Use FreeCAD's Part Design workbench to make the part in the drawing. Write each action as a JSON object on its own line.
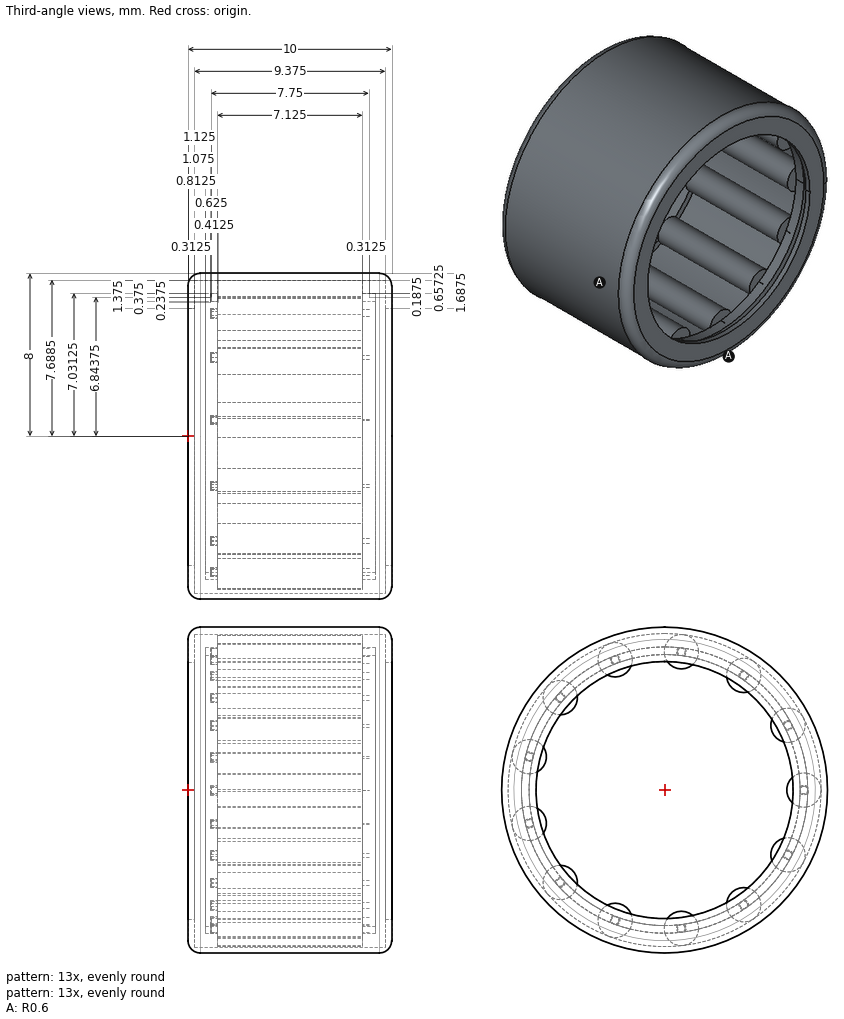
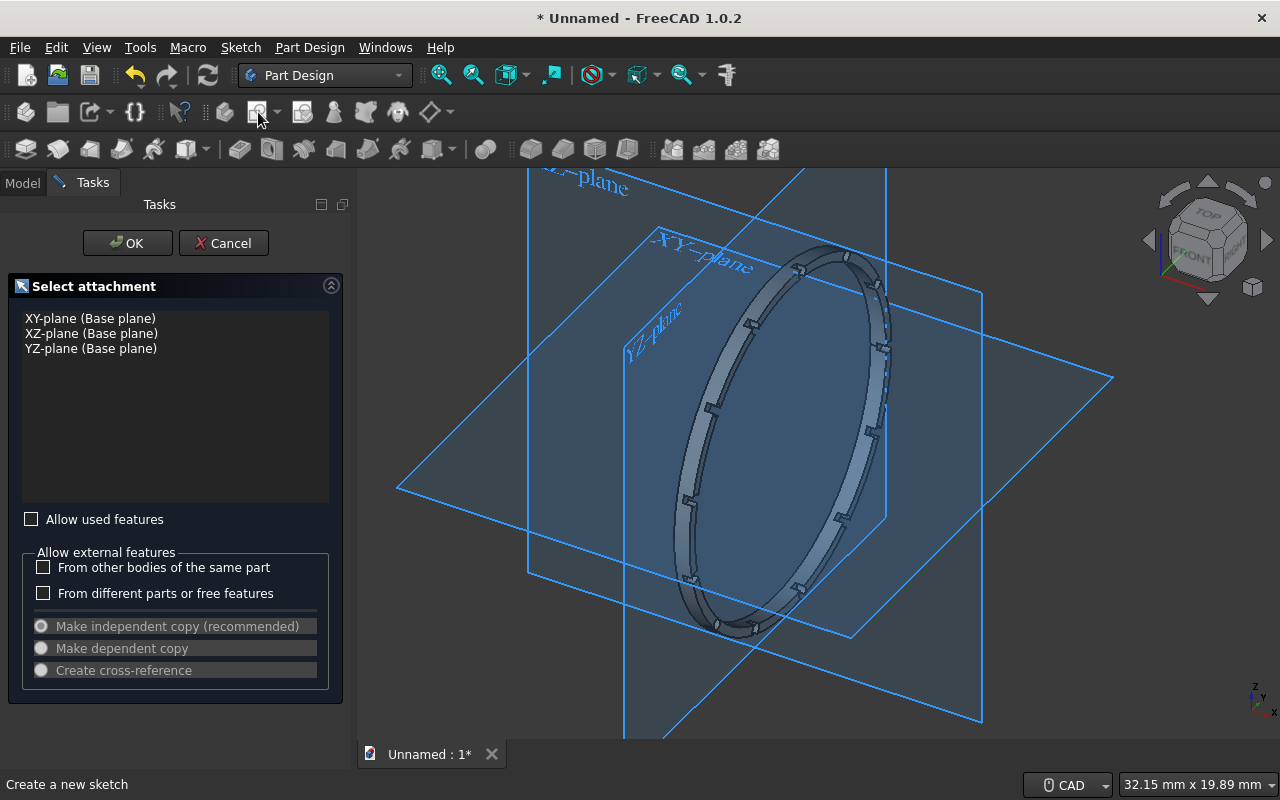
{"action": "left_click", "coordinate": [82, 318]}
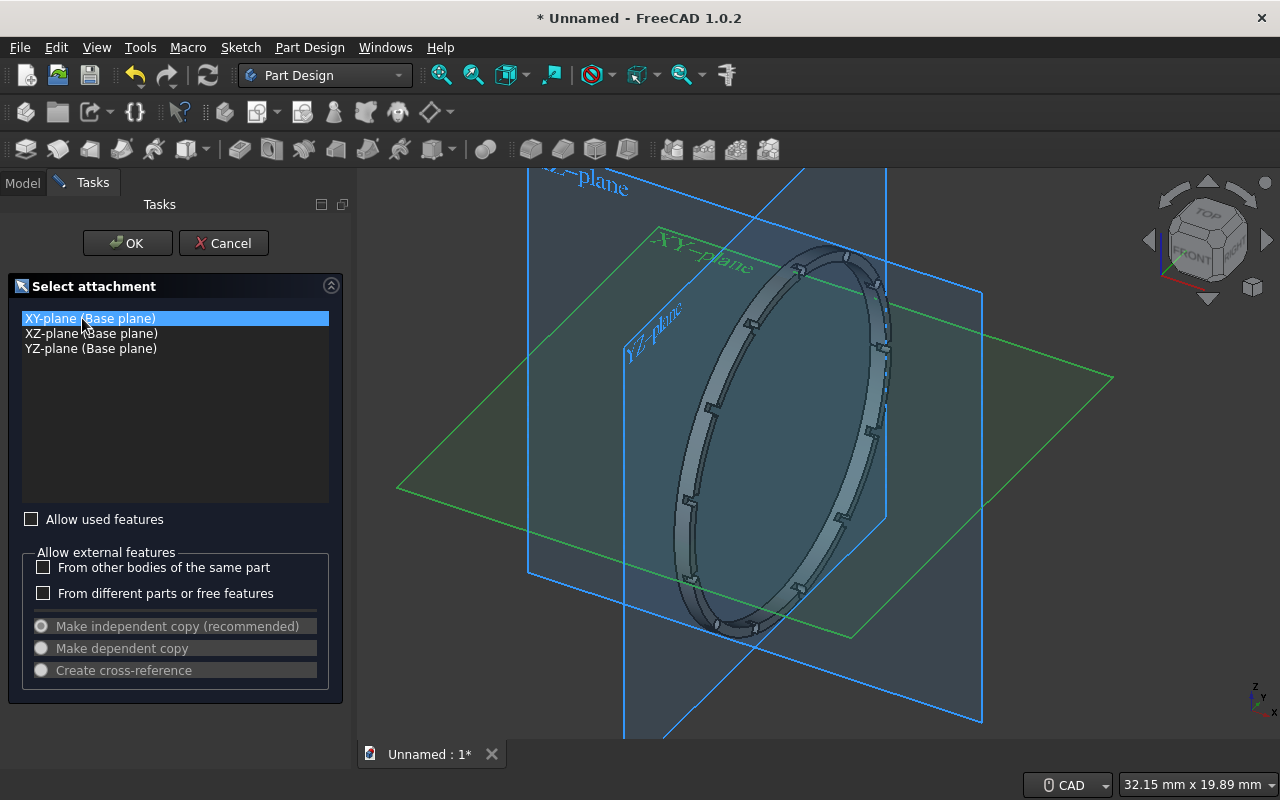
{"action": "left_click", "coordinate": [128, 243]}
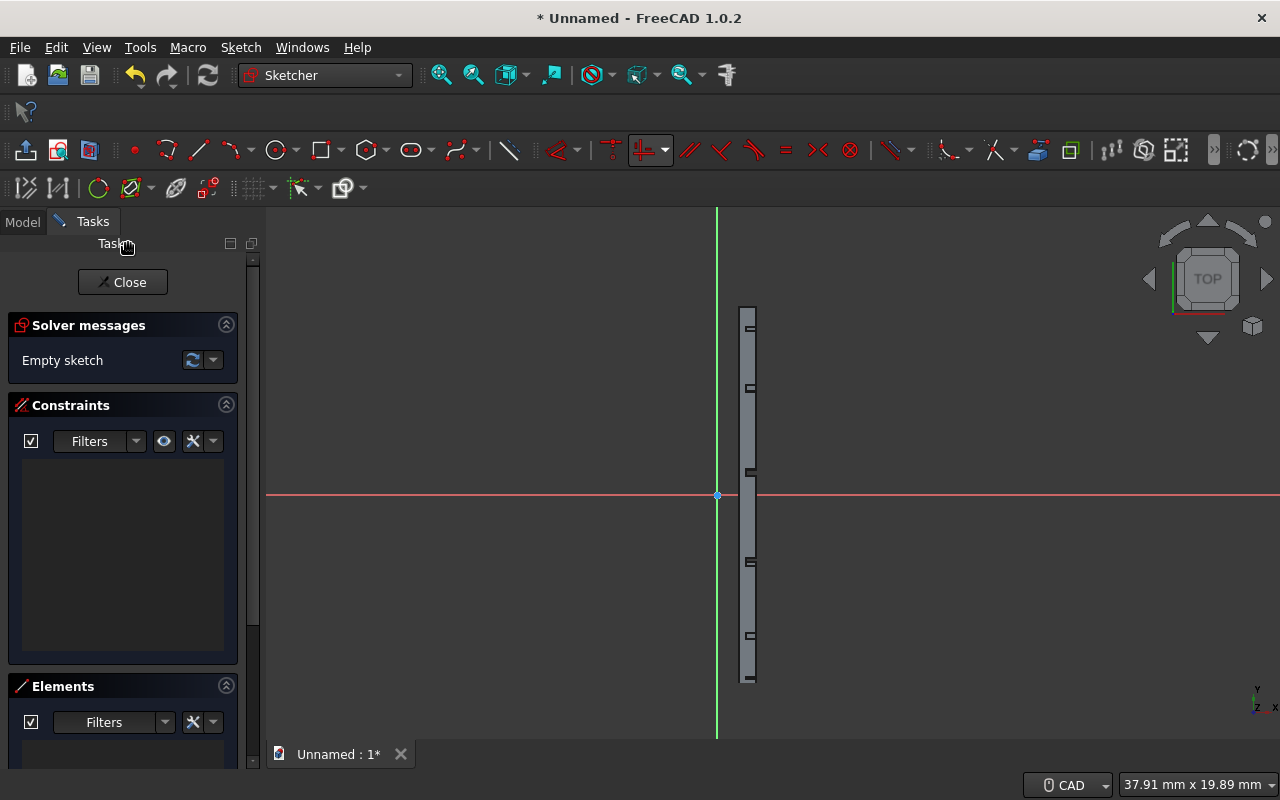
{"action": "left_click", "coordinate": [90, 150]}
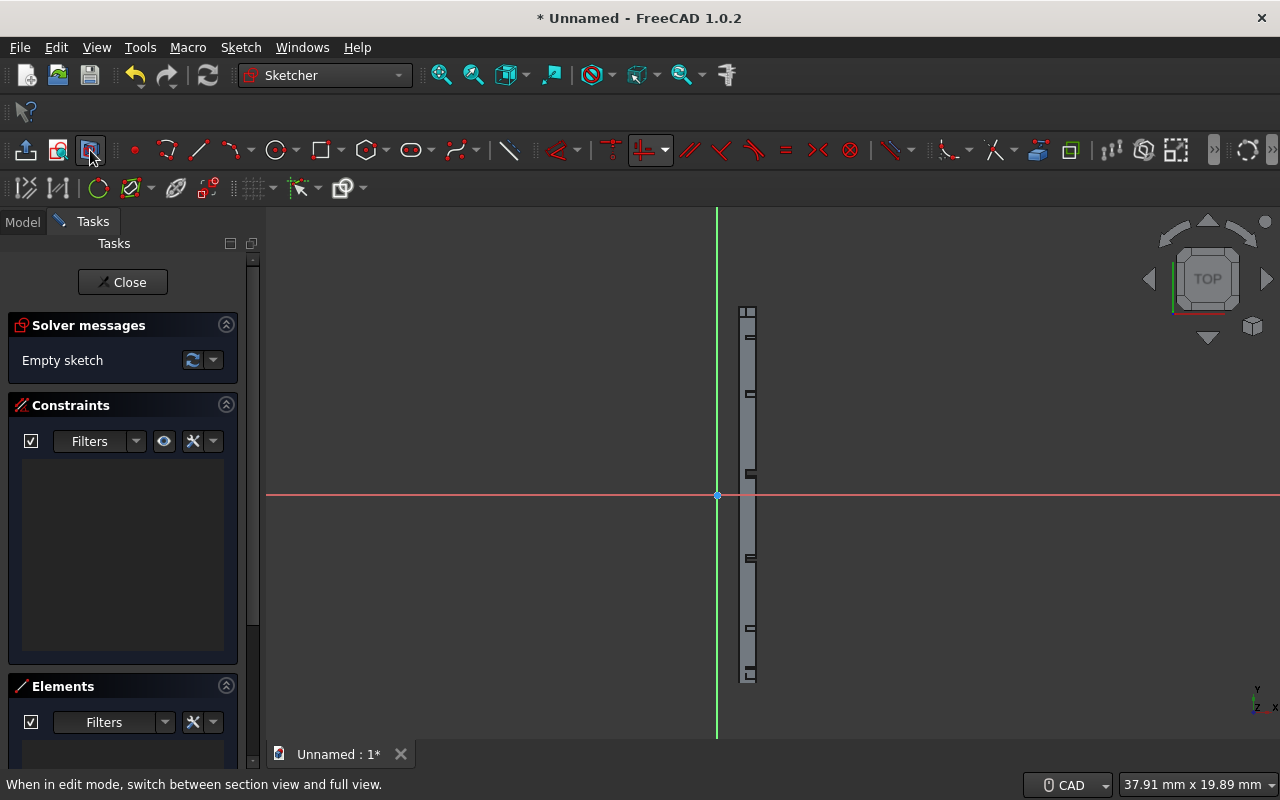
{"action": "scroll", "coordinate": [1115, 235], "scroll_direction": "up", "scroll_amount": 2}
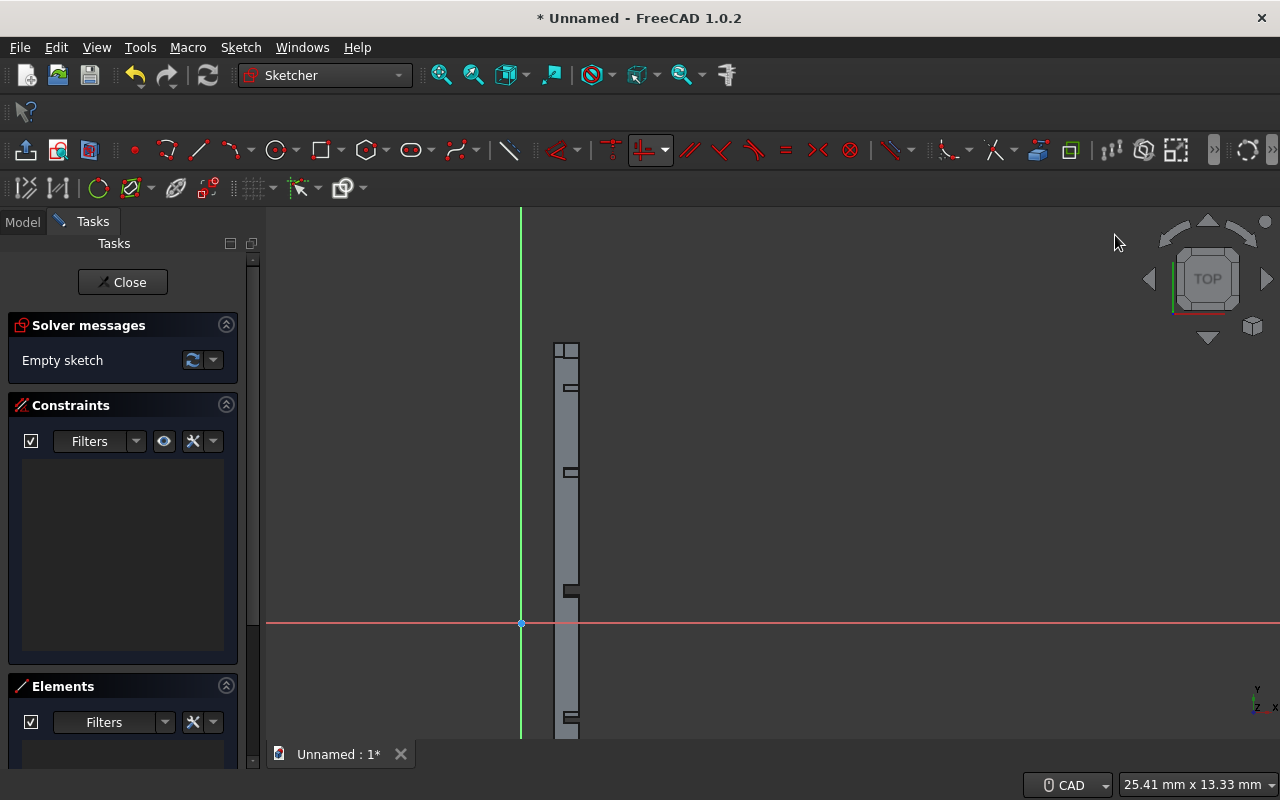
{"action": "left_click", "coordinate": [168, 150]}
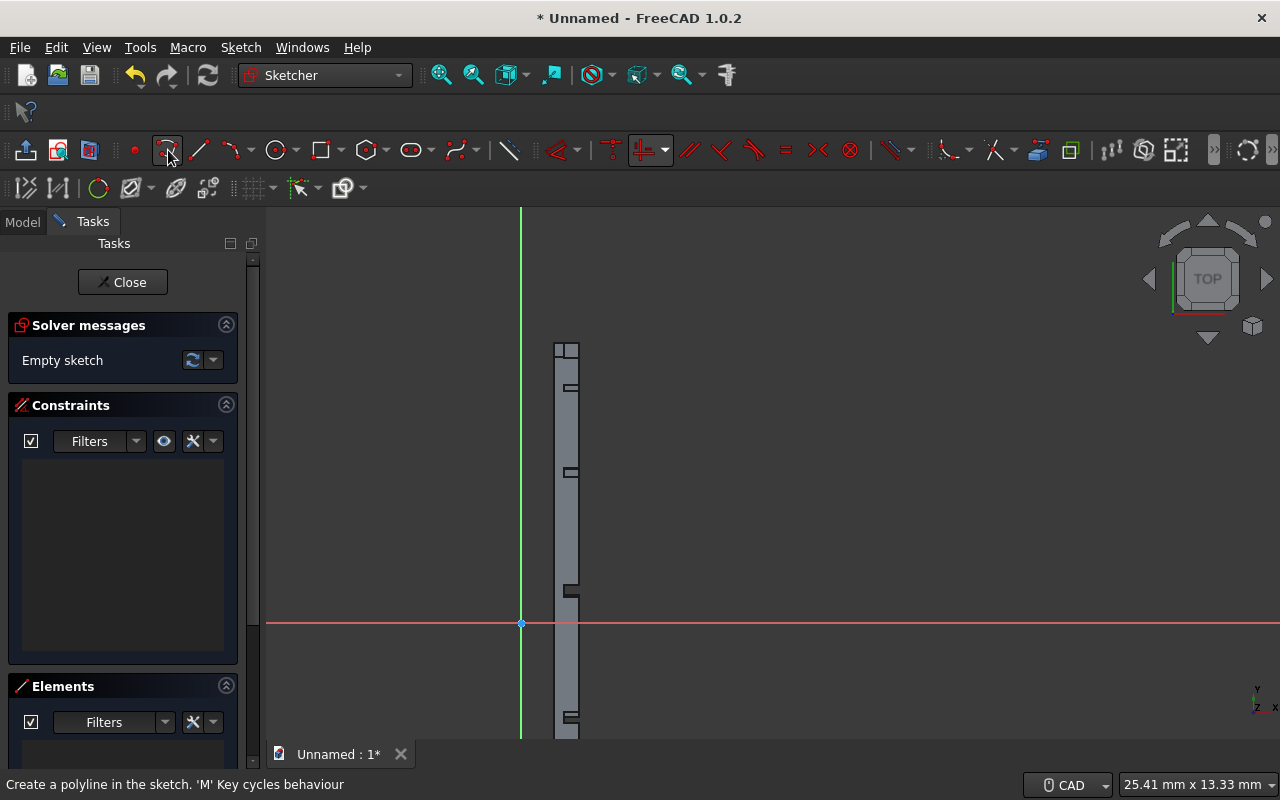
{"action": "left_click", "coordinate": [566, 350]}
{"action": "left_click", "coordinate": [875, 350]}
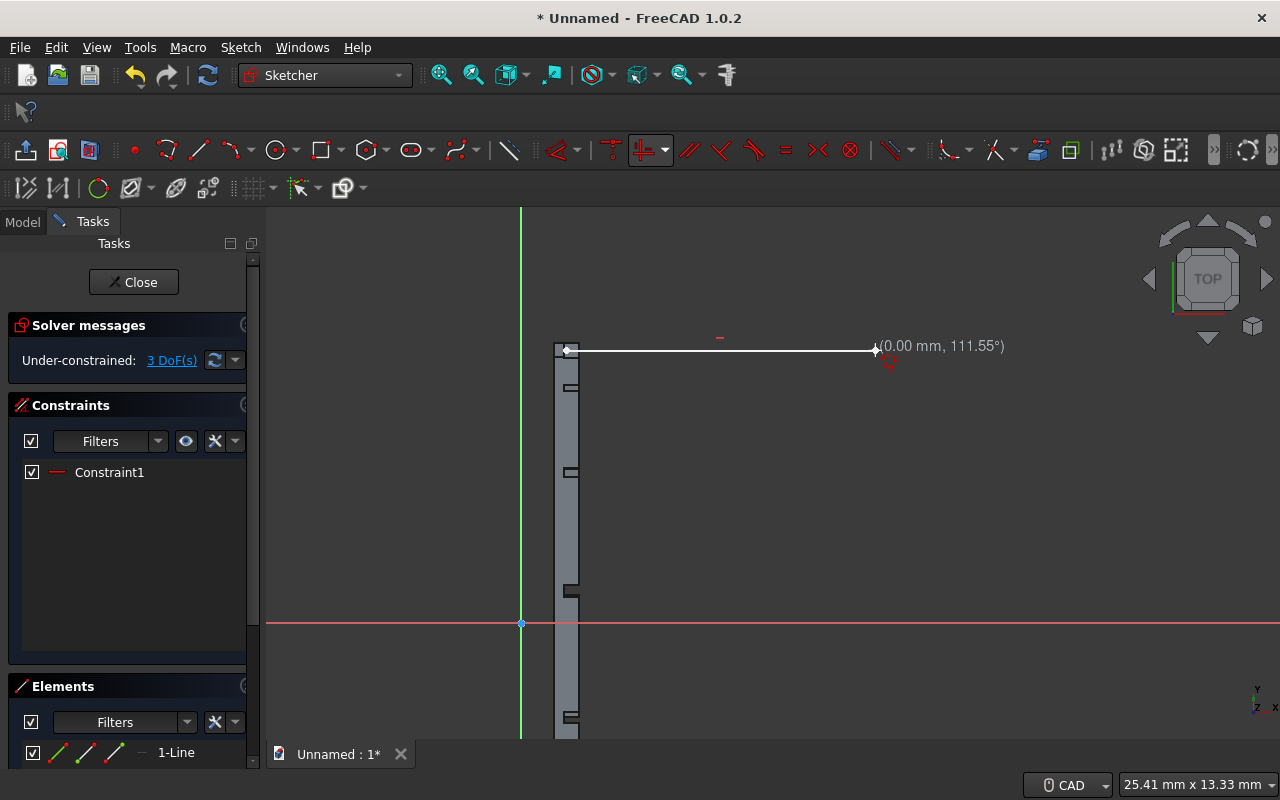
{"action": "scroll", "coordinate": [875, 343], "scroll_direction": "up", "scroll_amount": 4}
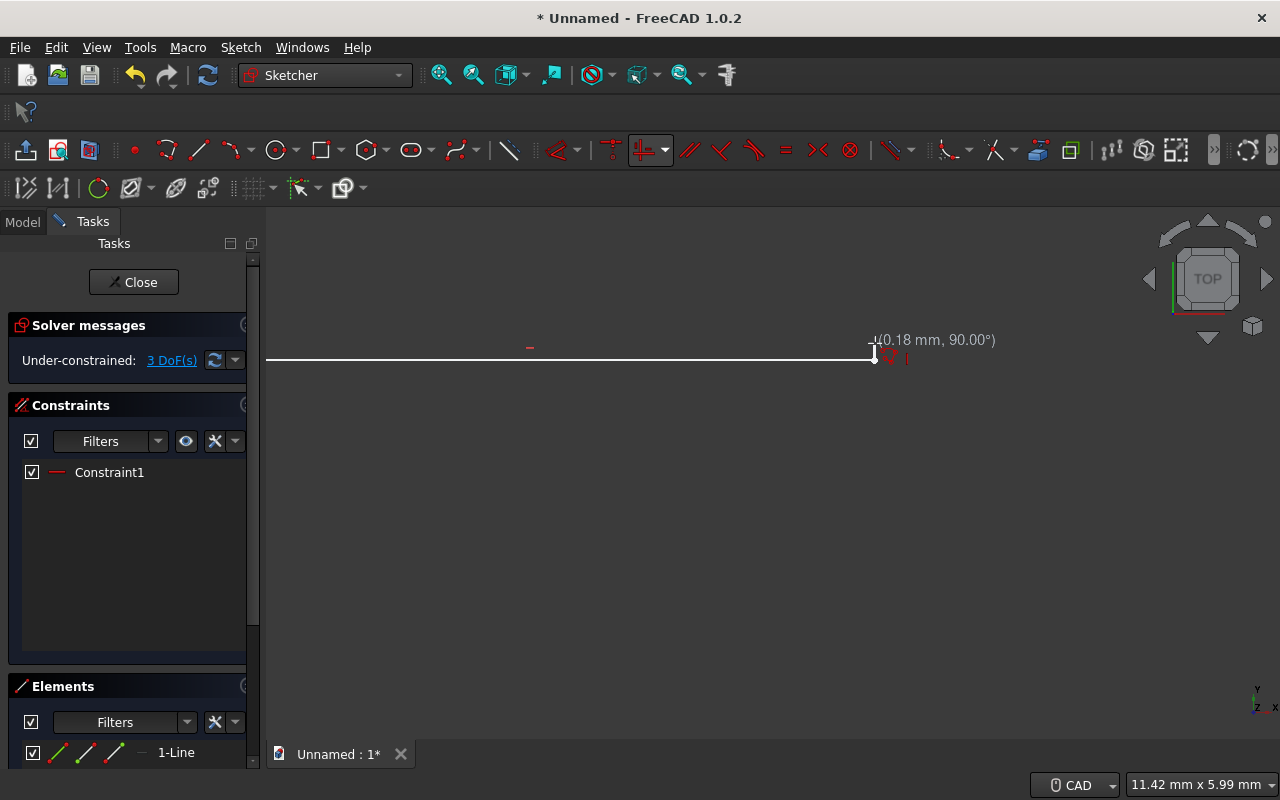
{"action": "left_click", "coordinate": [874, 342]}
{"action": "left_click", "coordinate": [847, 342]}
{"action": "left_click", "coordinate": [847, 283]}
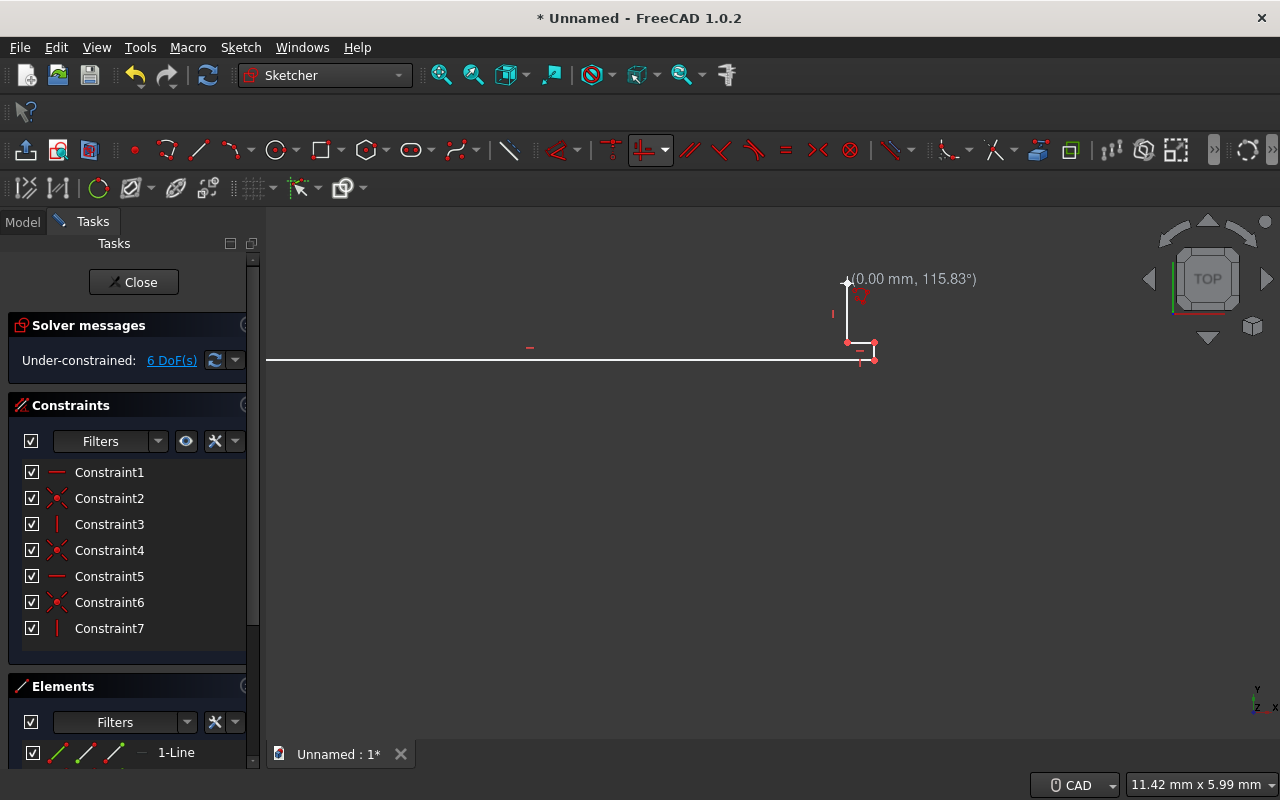
{"action": "scroll", "coordinate": [774, 349], "scroll_direction": "down", "scroll_amount": 4}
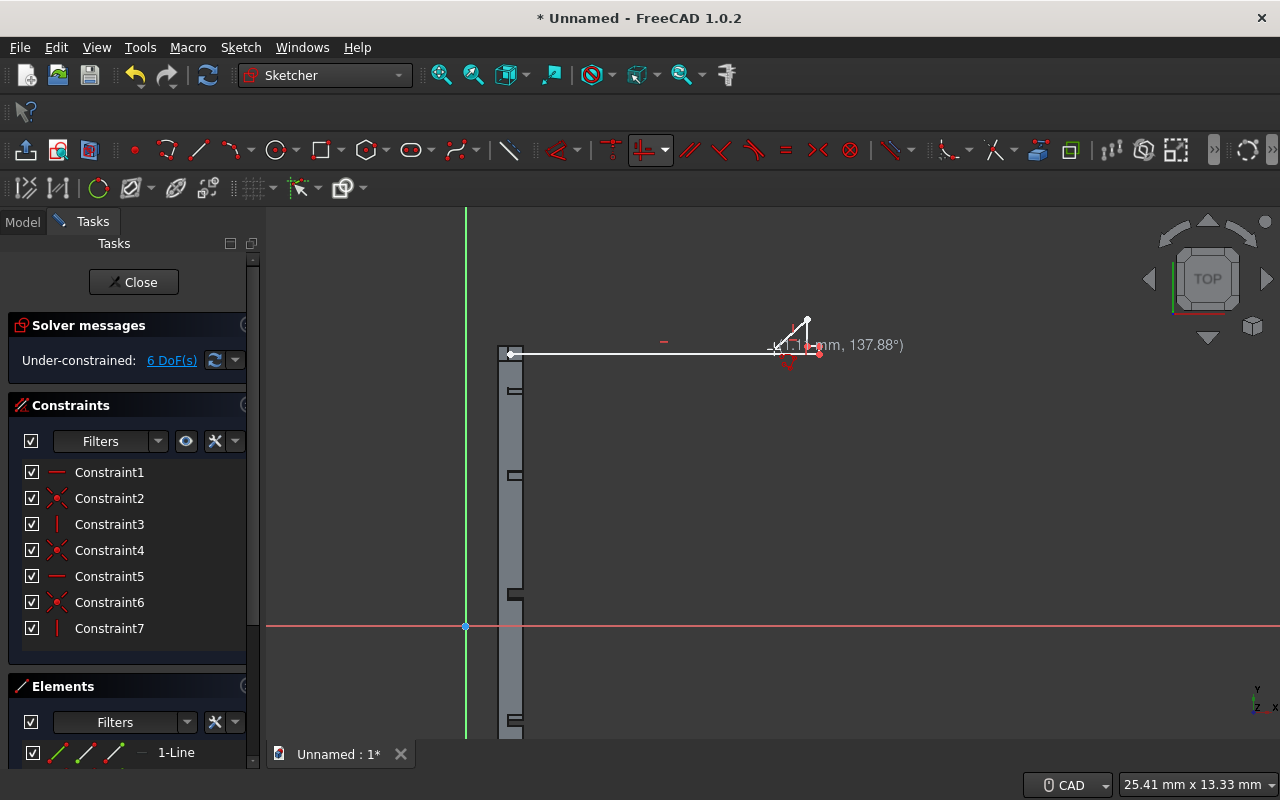
{"action": "left_click", "coordinate": [523, 319]}